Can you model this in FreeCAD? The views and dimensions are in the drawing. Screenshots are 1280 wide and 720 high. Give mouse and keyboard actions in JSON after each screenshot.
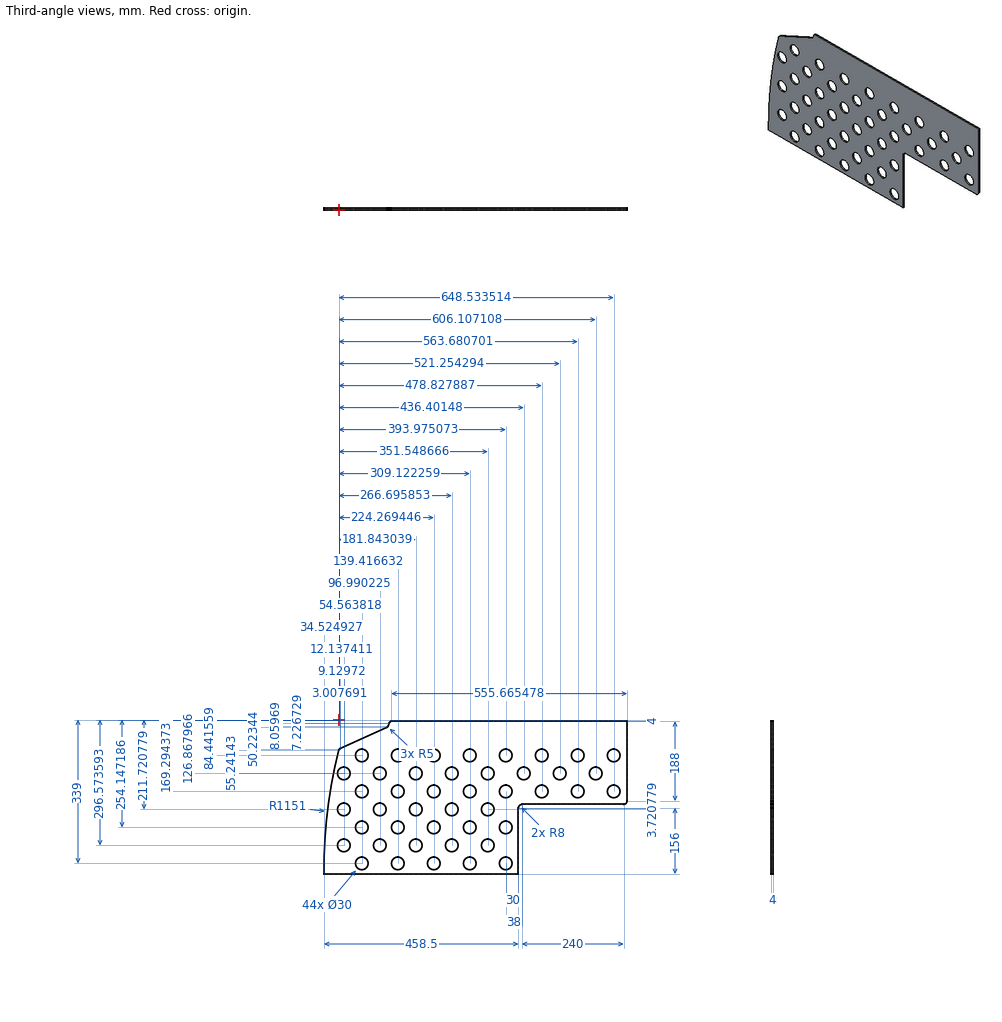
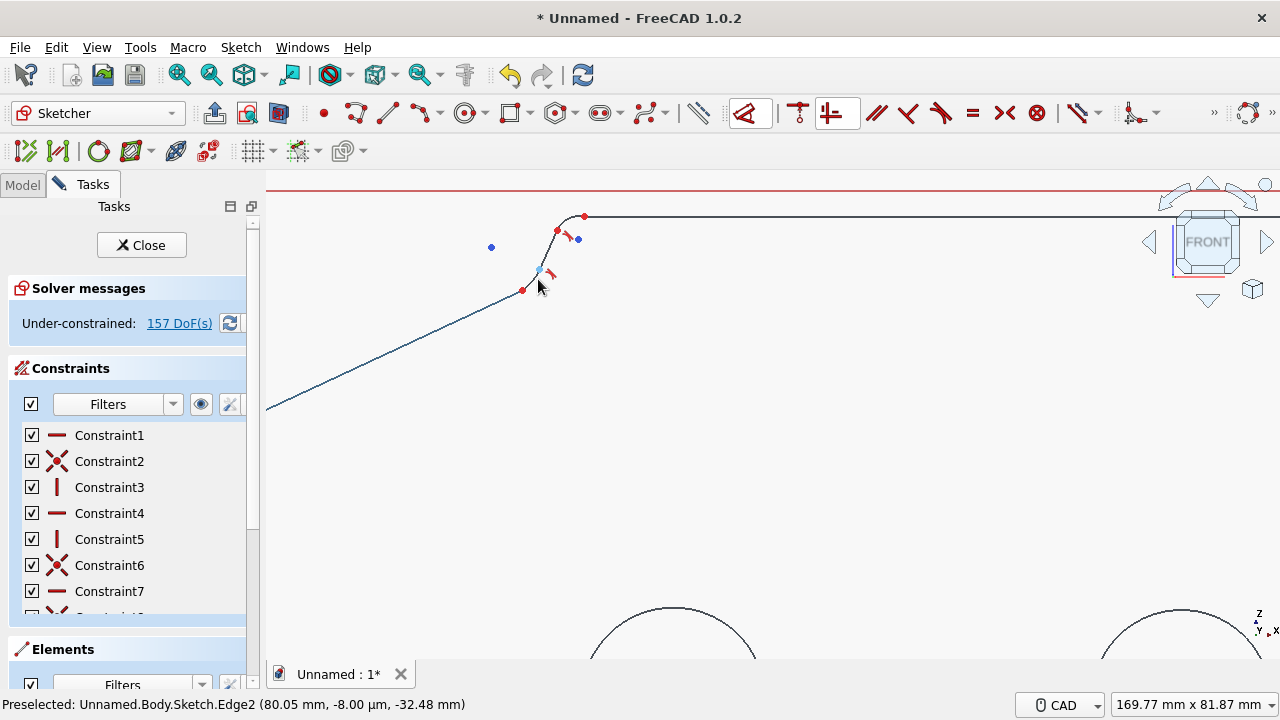
{"action": "left_click", "coordinate": [533, 281]}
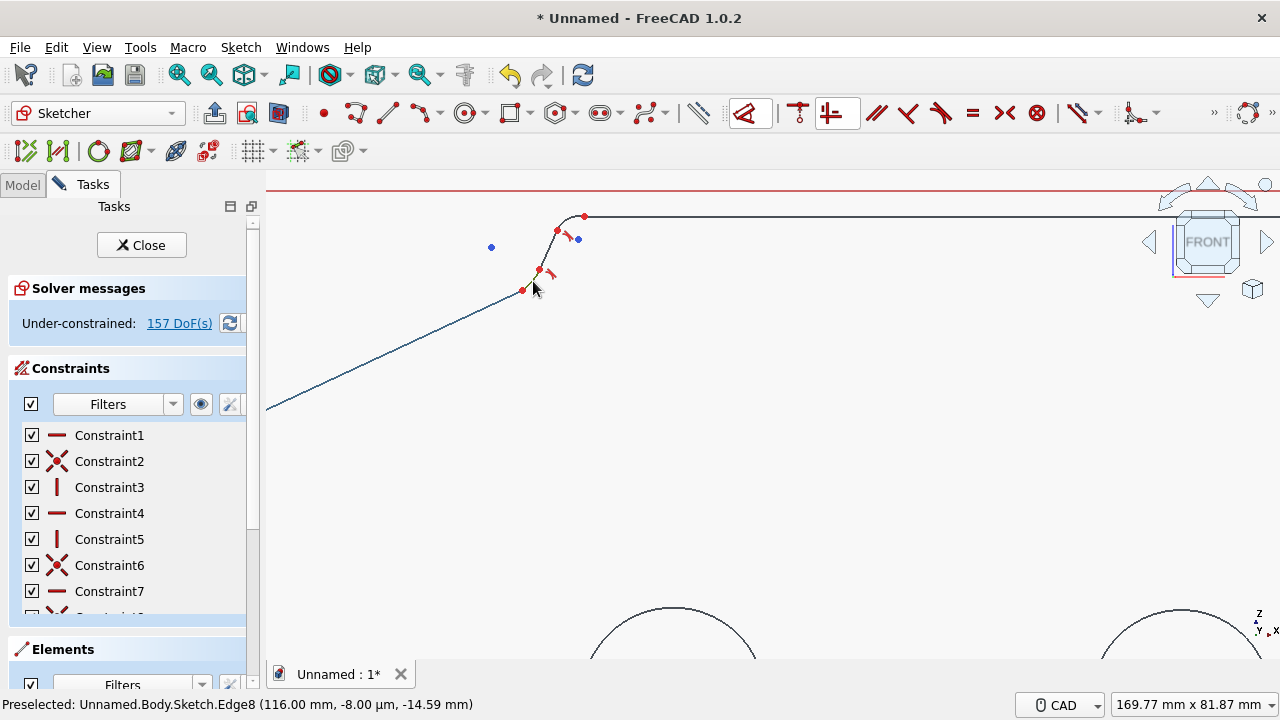
{"action": "left_click", "coordinate": [942, 114]}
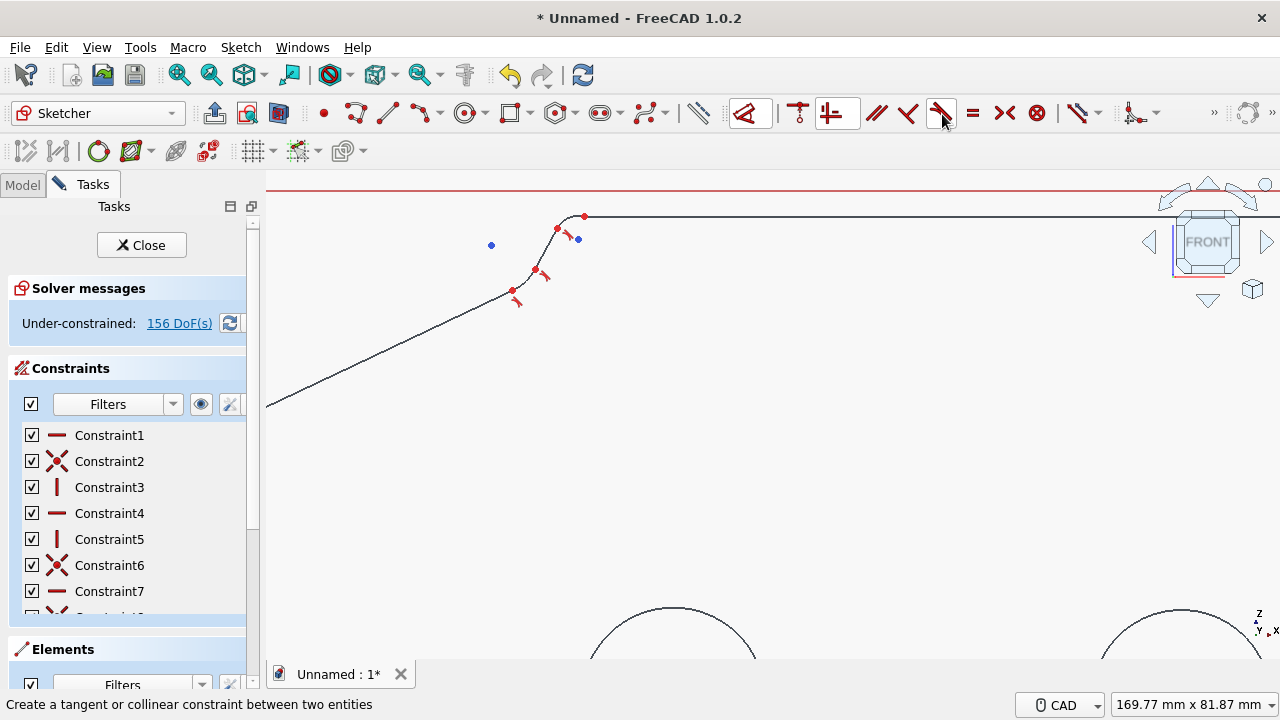
{"action": "scroll", "coordinate": [538, 279], "scroll_direction": "down", "scroll_amount": 10}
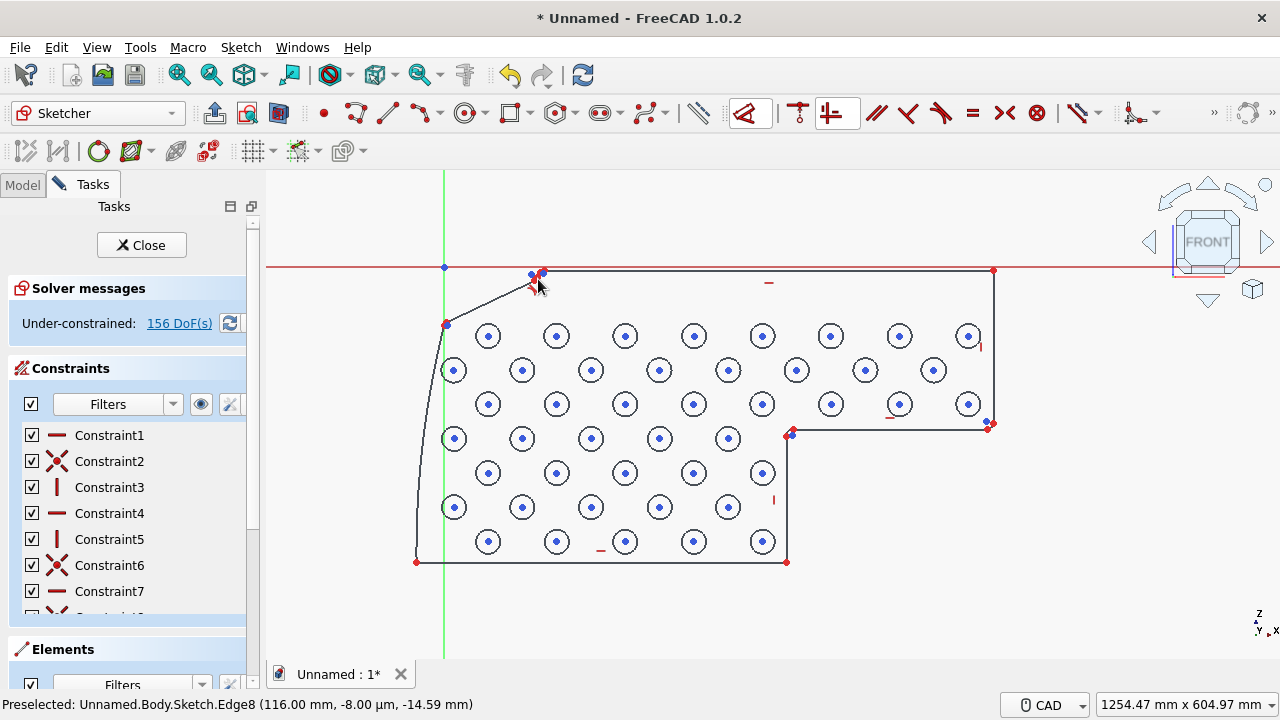
{"action": "left_click", "coordinate": [508, 293]}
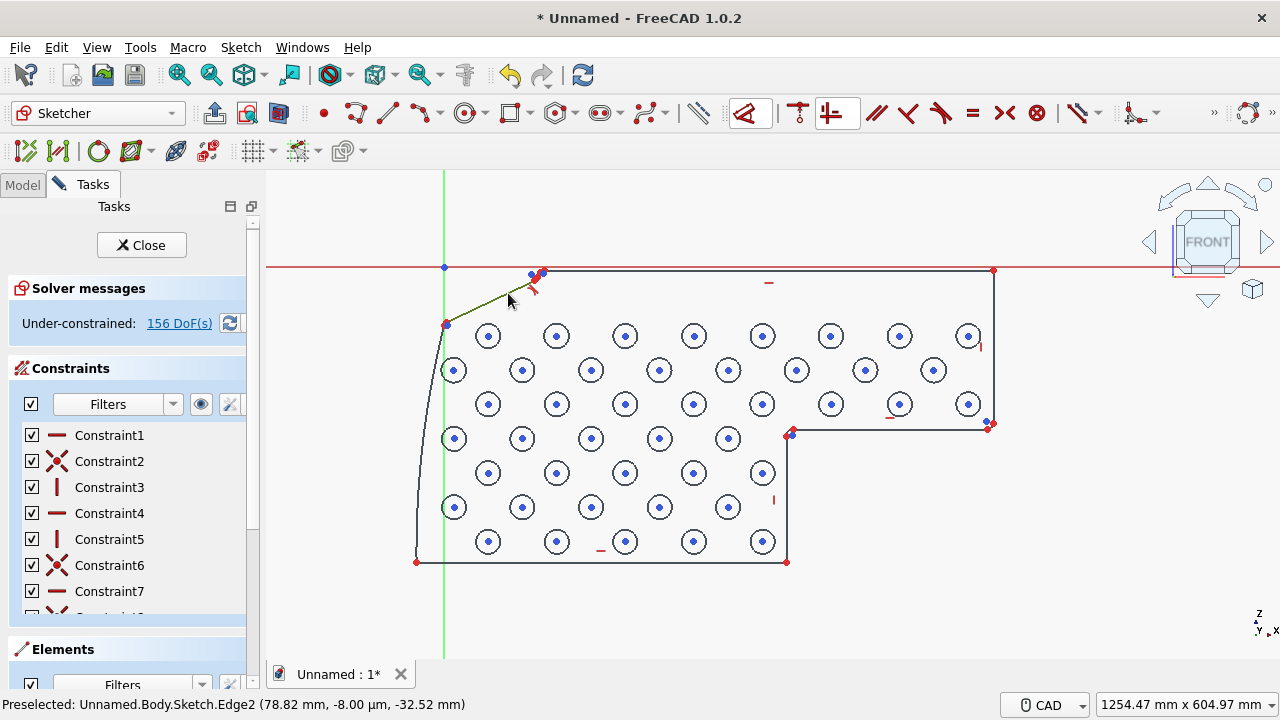
{"action": "scroll", "coordinate": [445, 324], "scroll_direction": "up", "scroll_amount": 11}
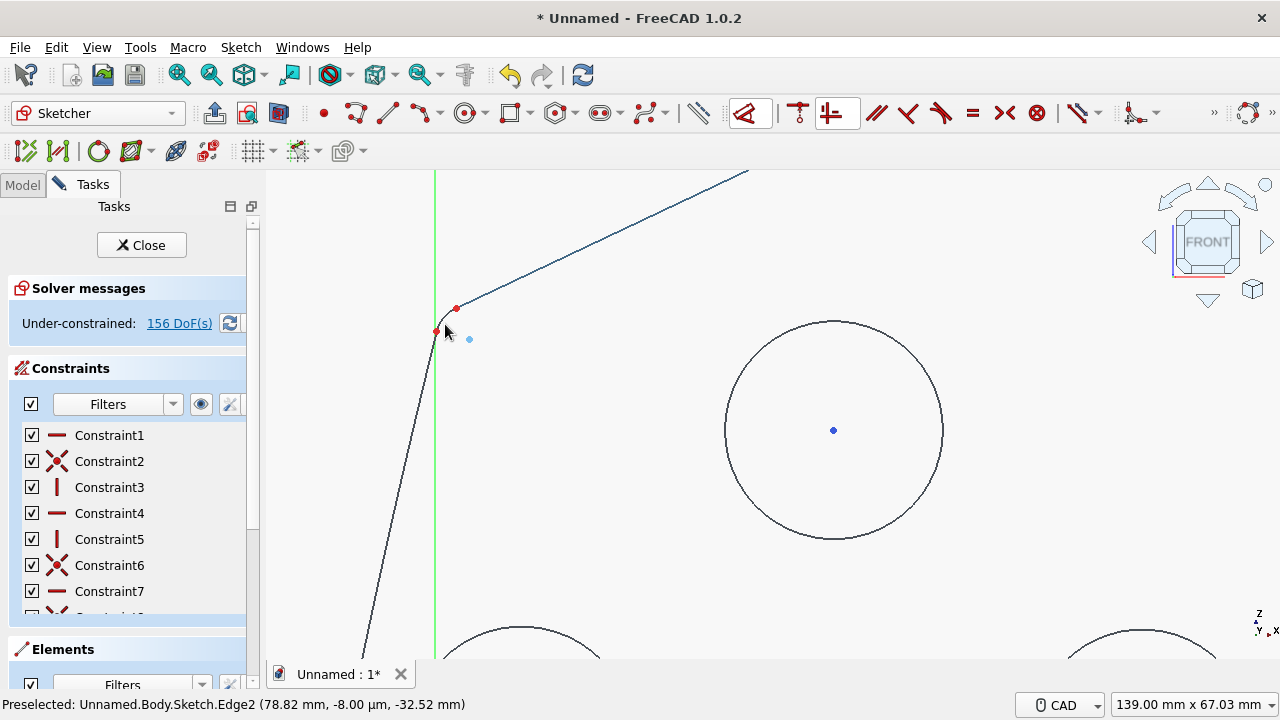
{"action": "left_click", "coordinate": [444, 318]}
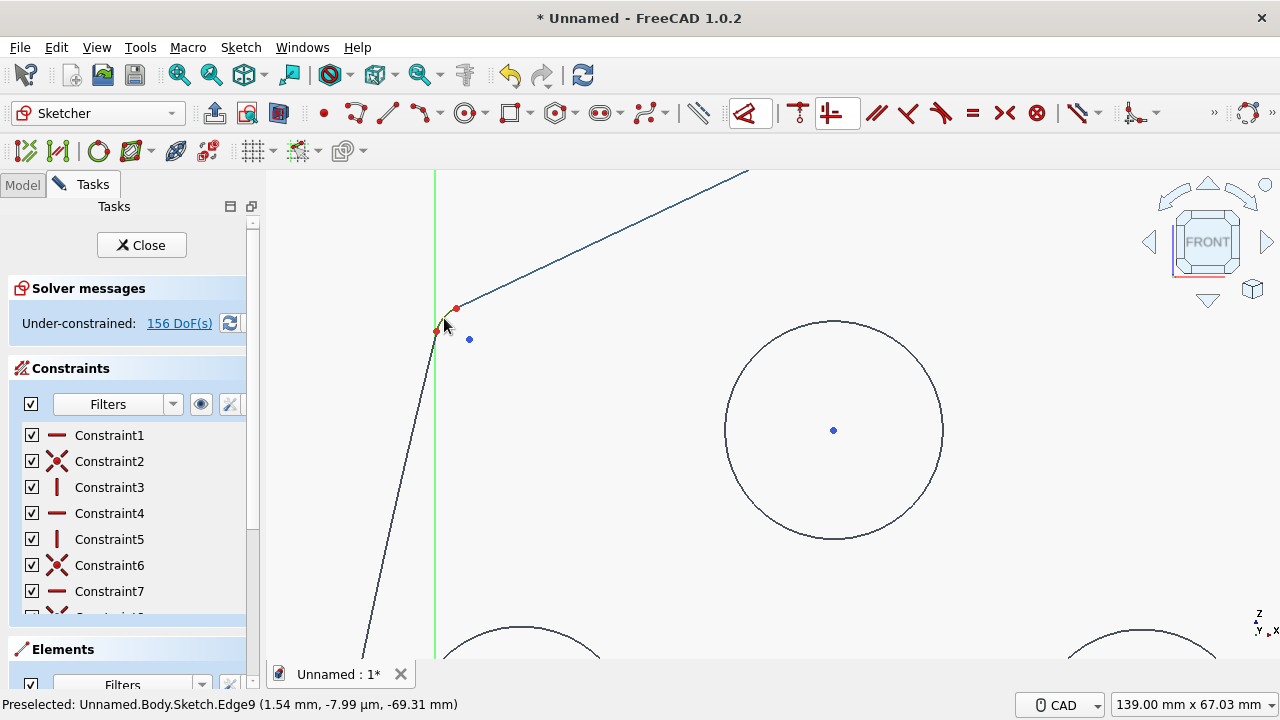
{"action": "left_click", "coordinate": [942, 114]}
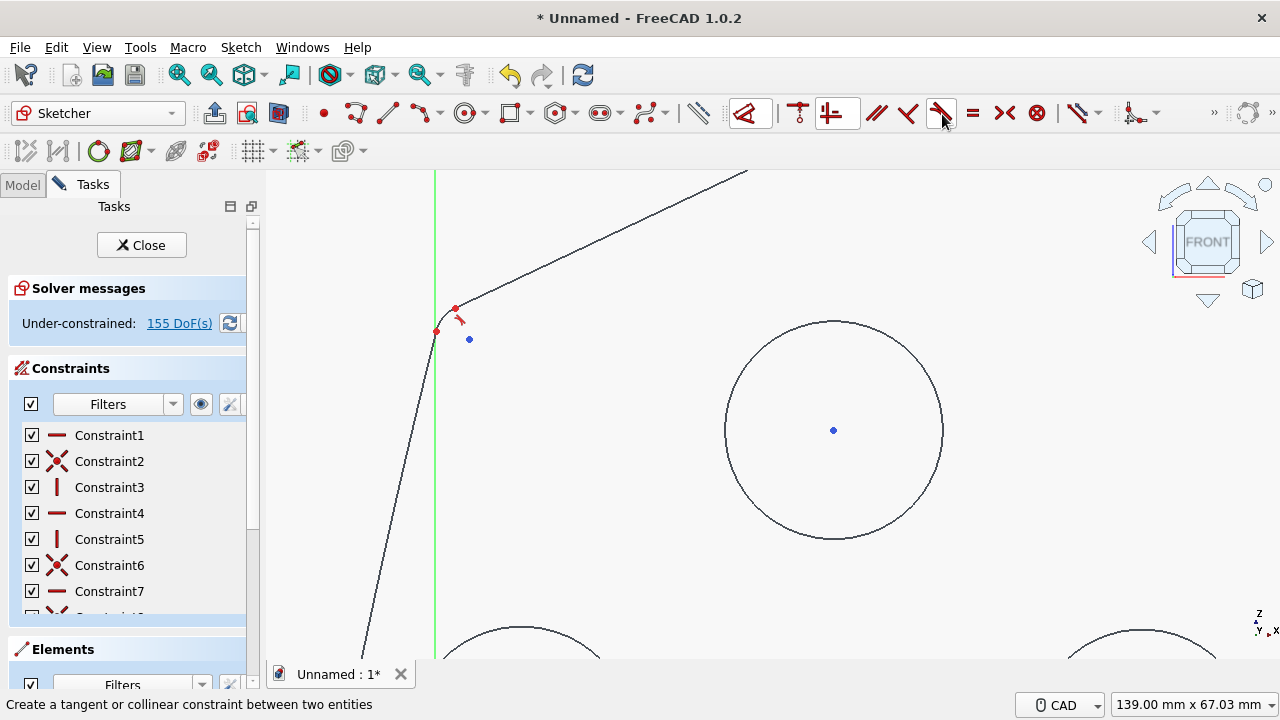
{"action": "scroll", "coordinate": [445, 324], "scroll_direction": "down", "scroll_amount": 11}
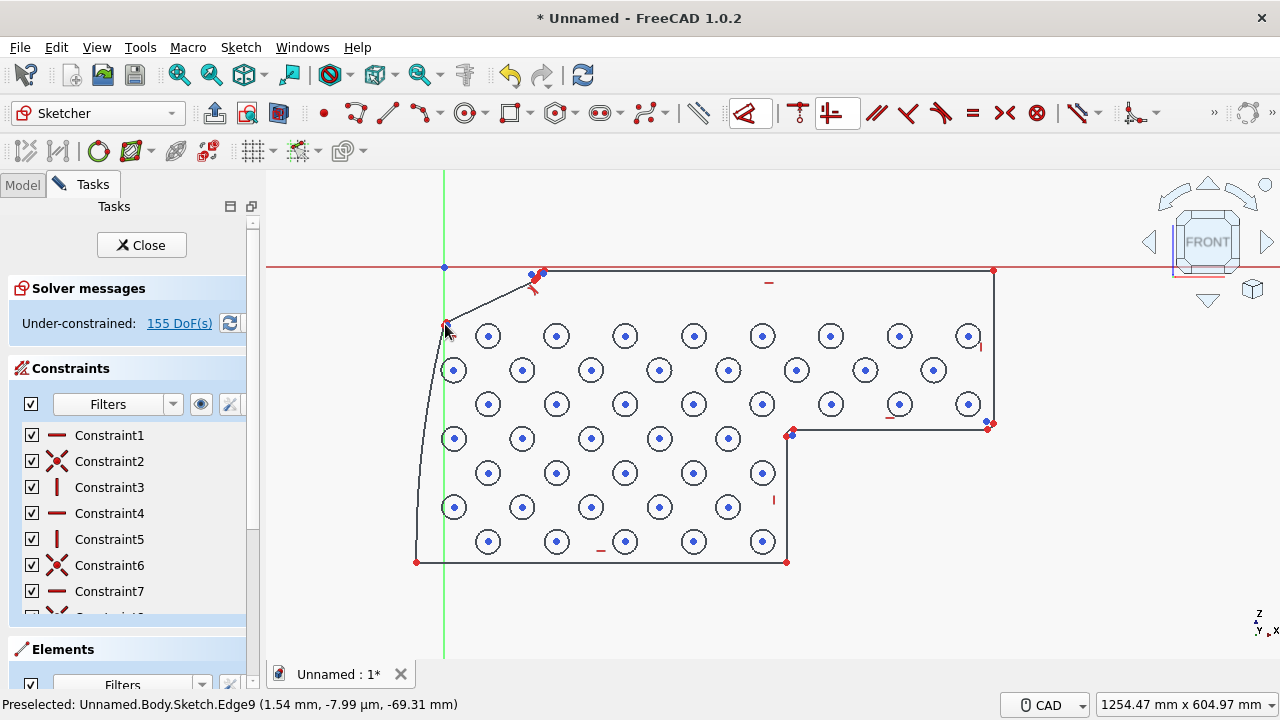
{"action": "left_click", "coordinate": [787, 525]}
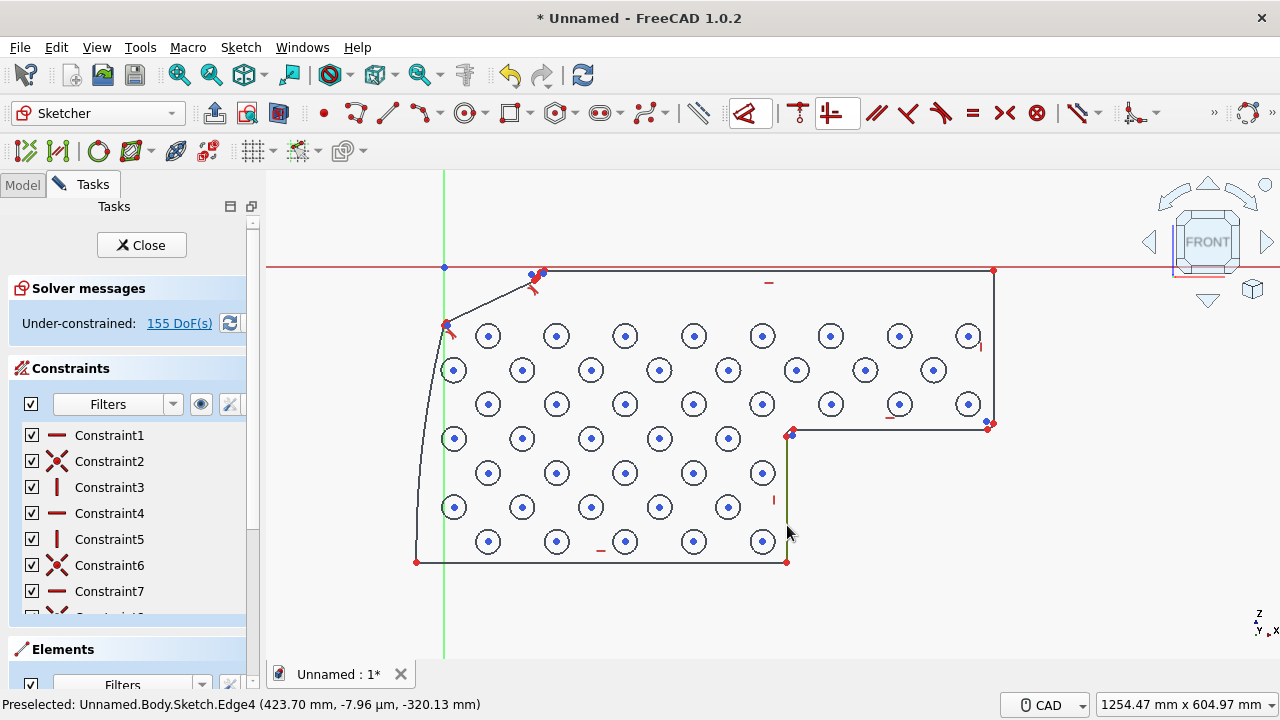
{"action": "scroll", "coordinate": [788, 431], "scroll_direction": "up", "scroll_amount": 5}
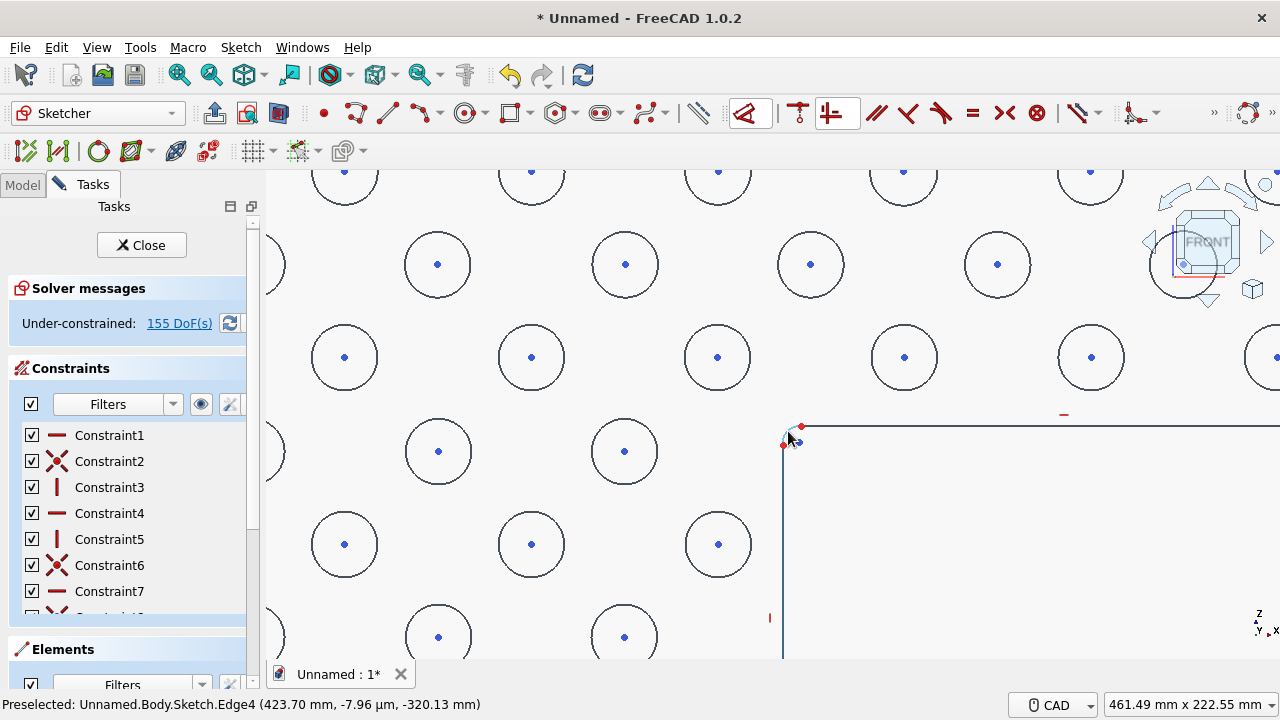
{"action": "left_click", "coordinate": [787, 431]}